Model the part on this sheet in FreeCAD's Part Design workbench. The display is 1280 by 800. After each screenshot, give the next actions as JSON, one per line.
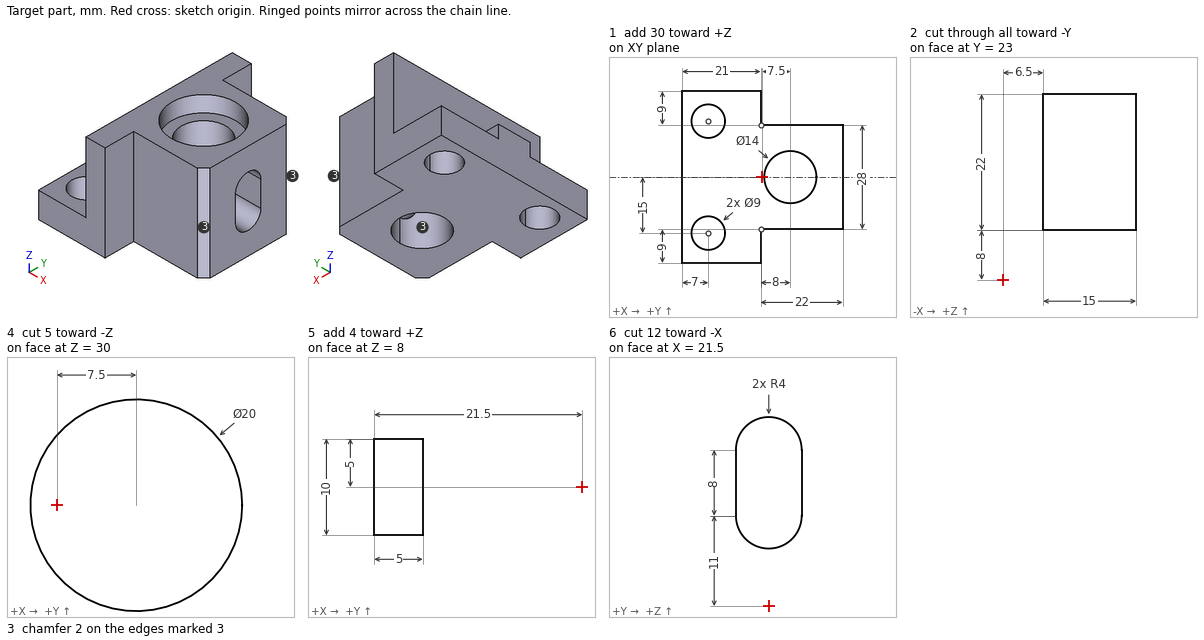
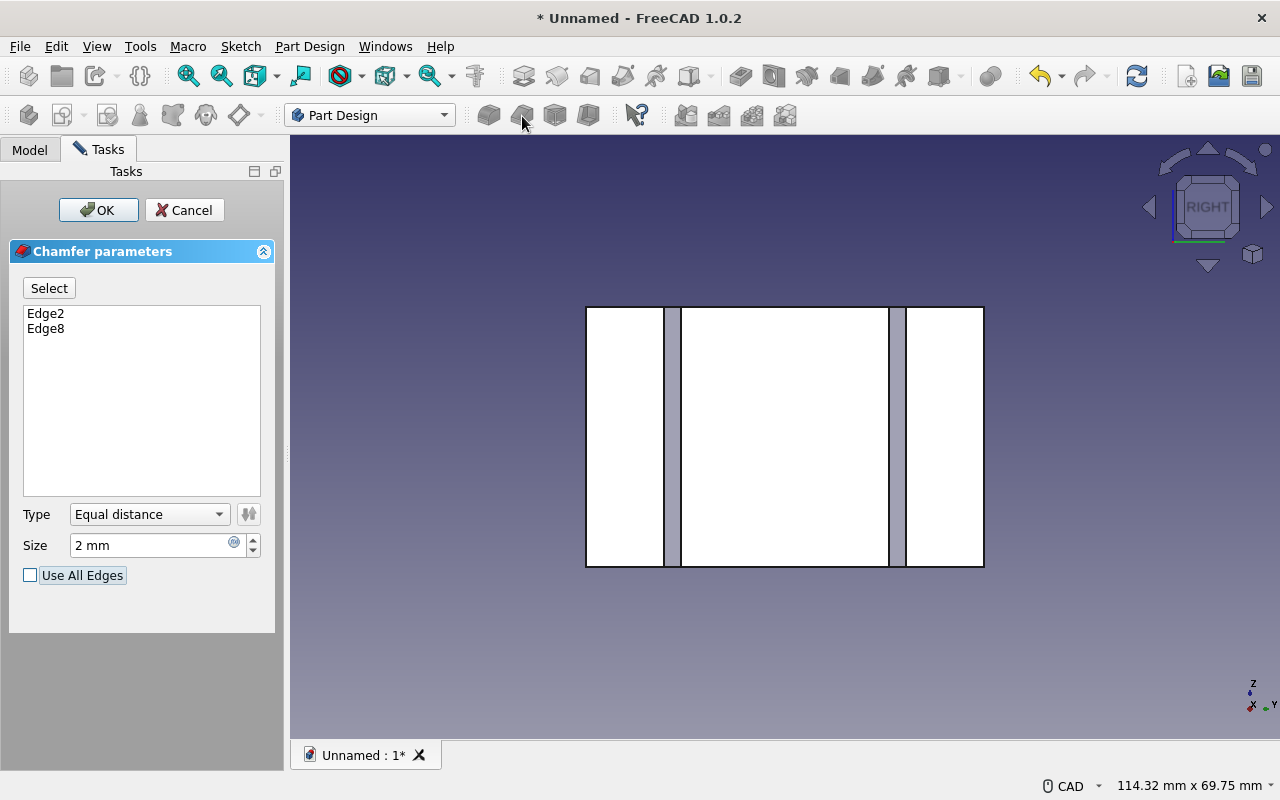
{"action": "left_click", "coordinate": [99, 210]}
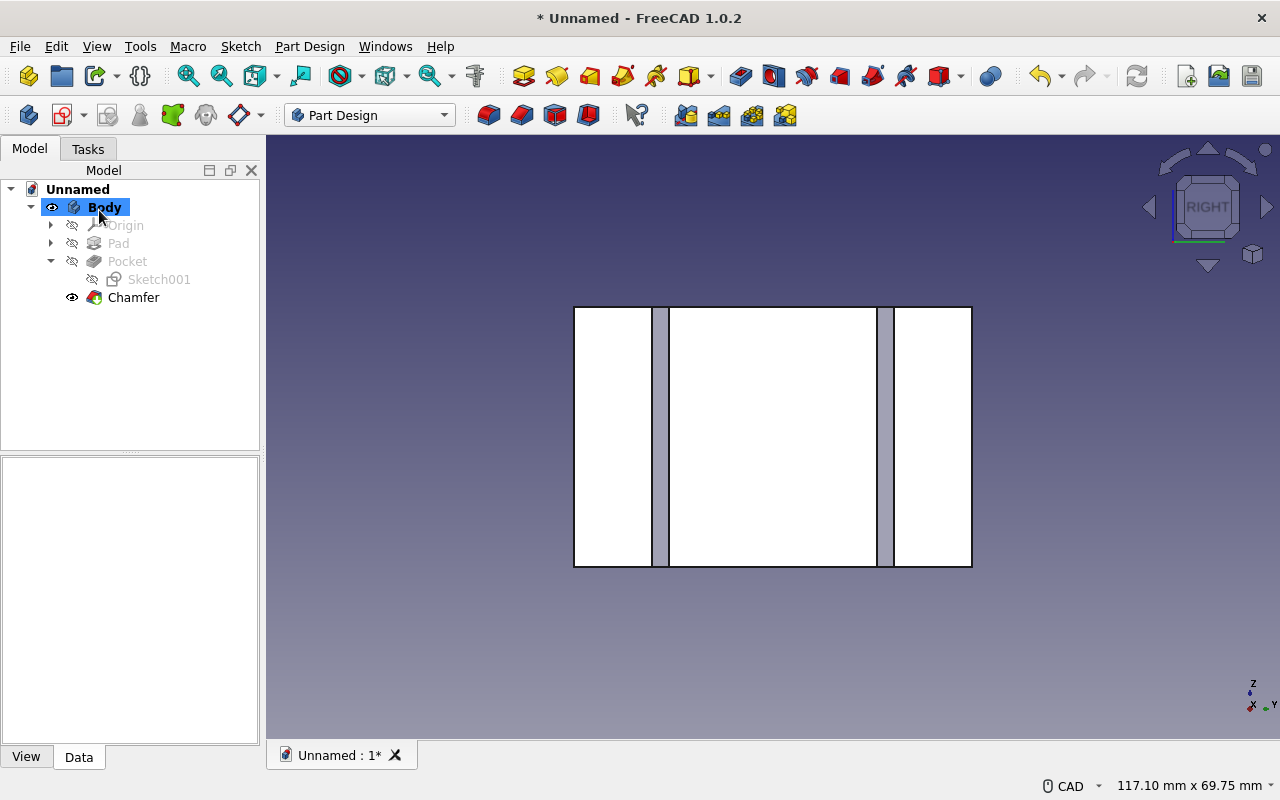
{"action": "key", "text": "v f"}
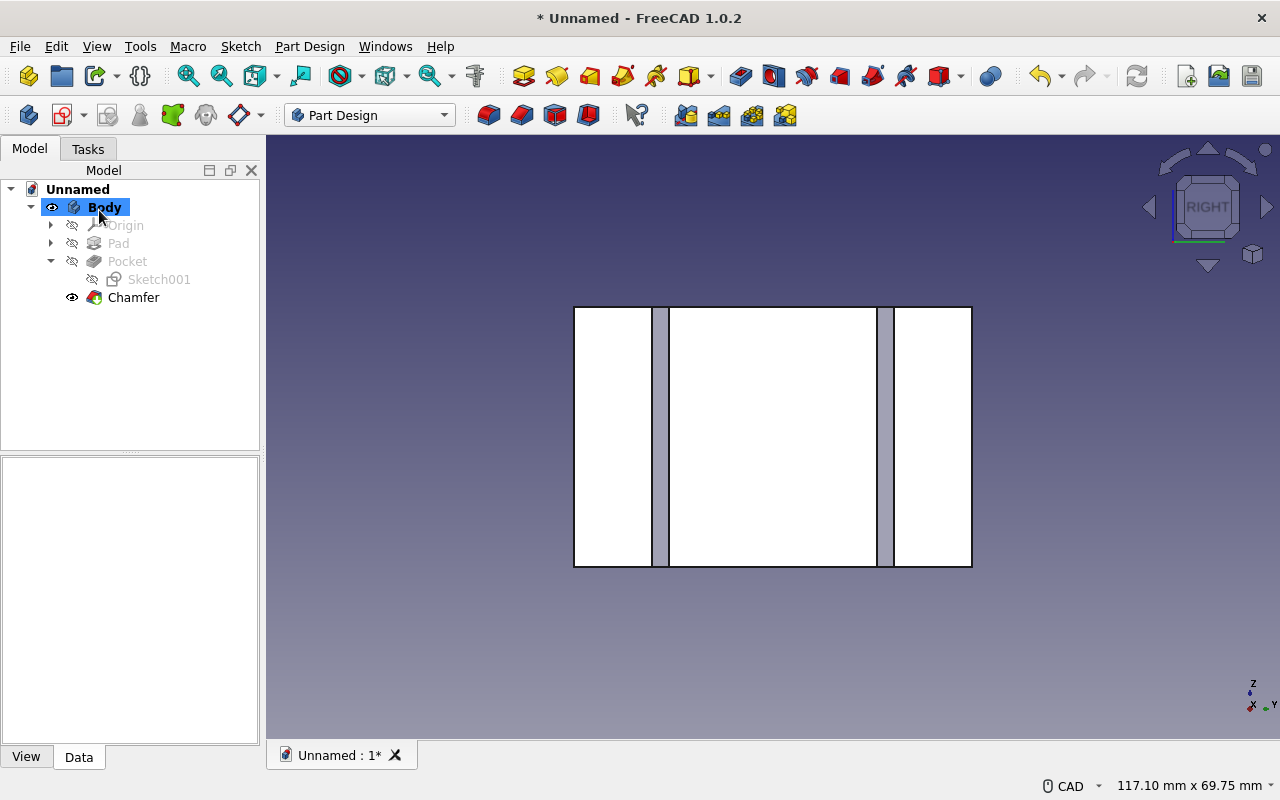
{"action": "key", "text": "0"}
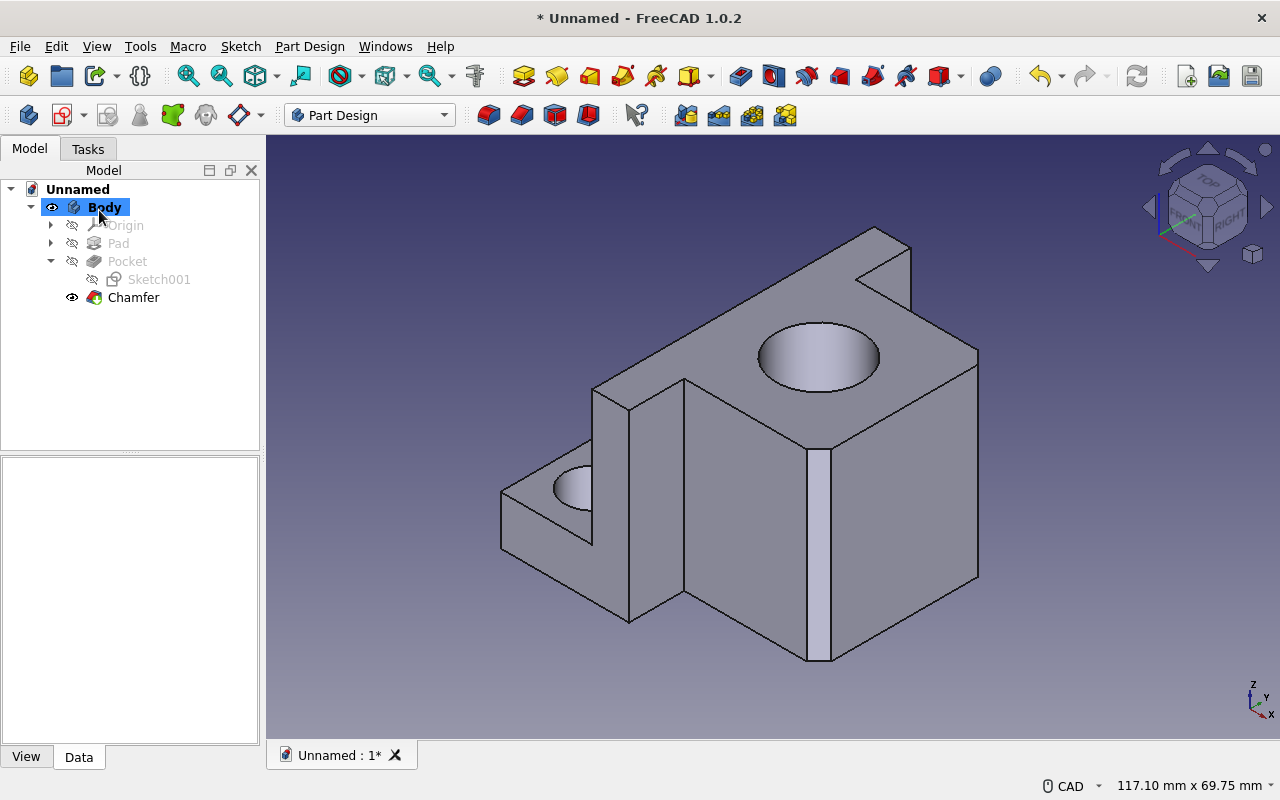
{"action": "left_click", "coordinate": [908, 362]}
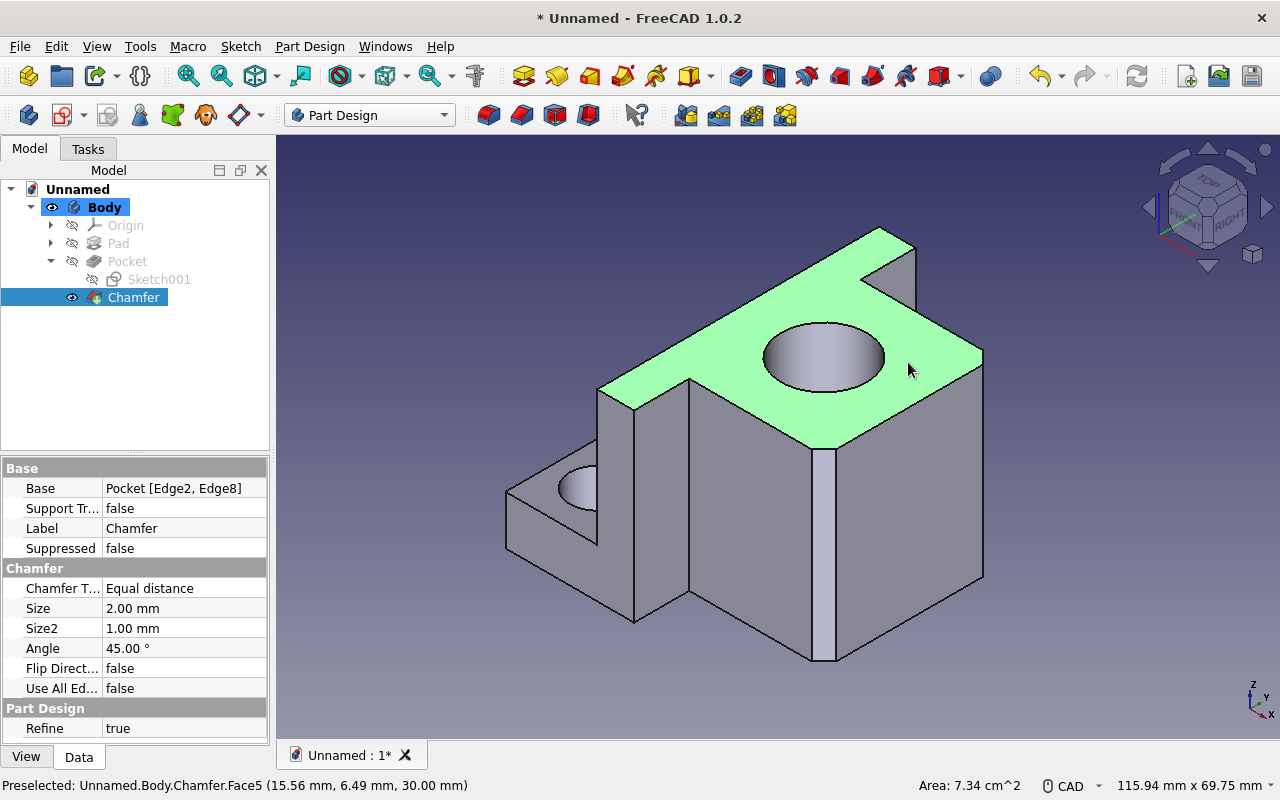
{"action": "left_click", "coordinate": [62, 116]}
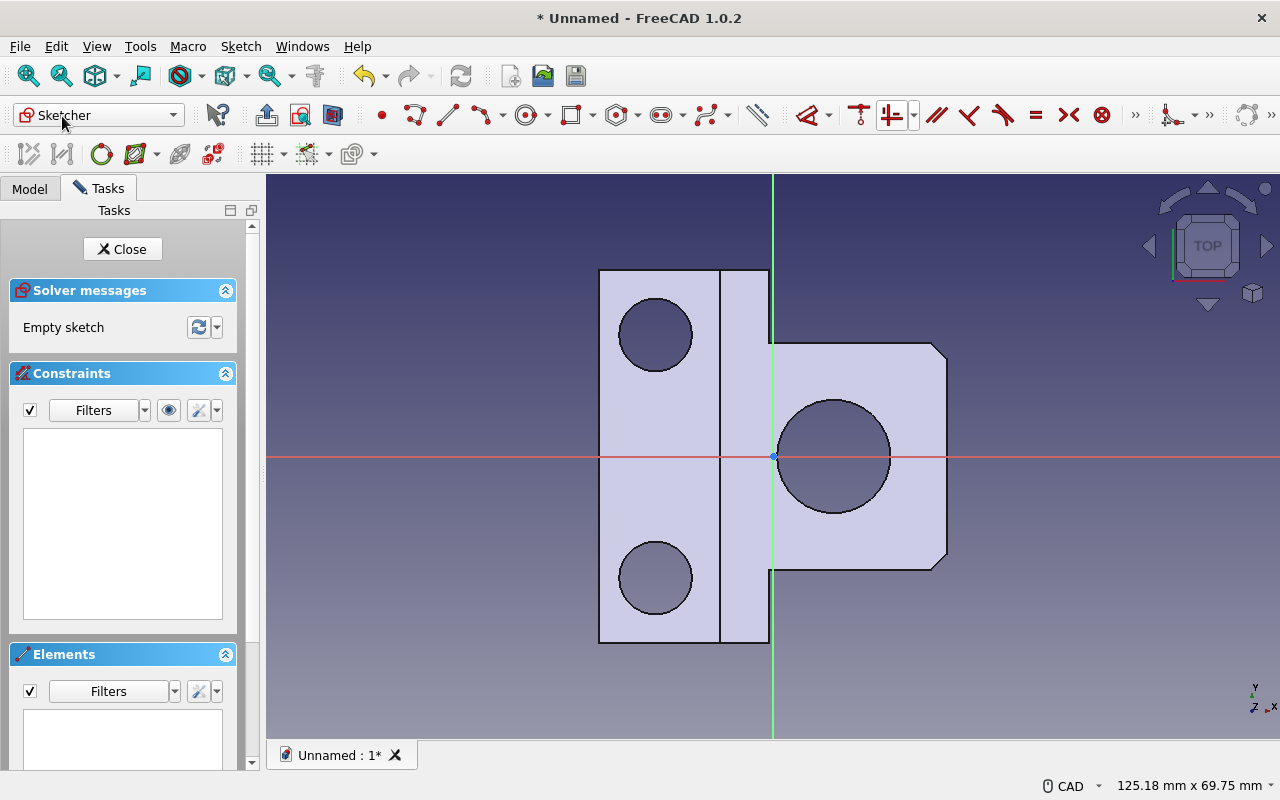
{"action": "scroll", "coordinate": [939, 456], "scroll_direction": "up", "scroll_amount": 4}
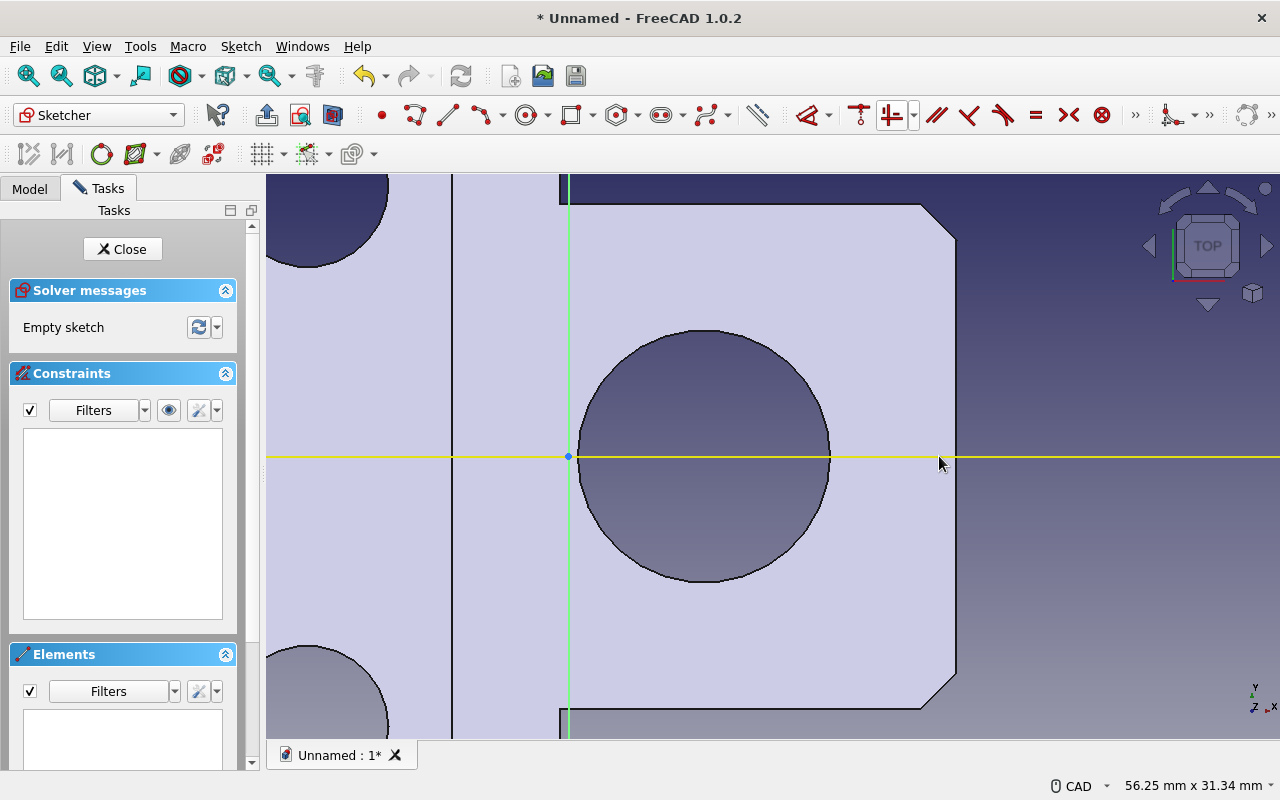
{"action": "key", "text": "g c"}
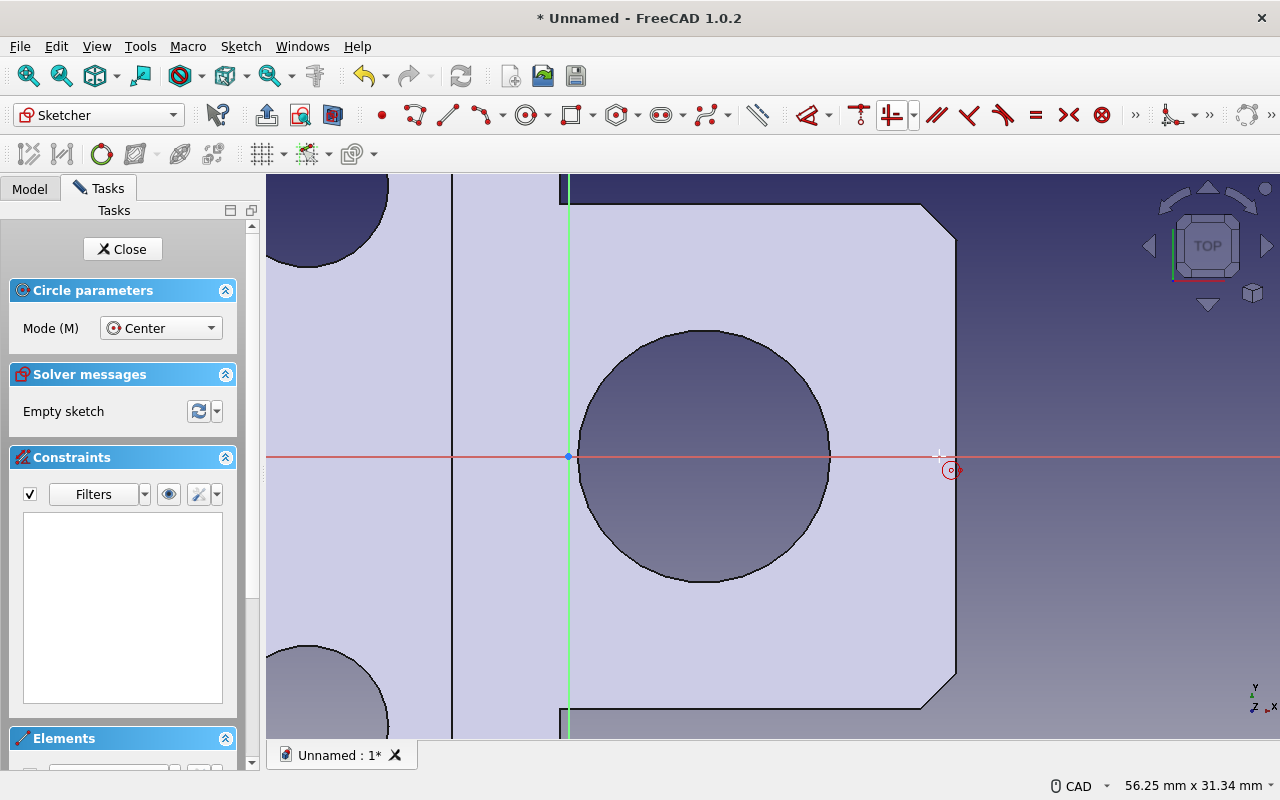
{"action": "left_click", "coordinate": [704, 456]}
{"action": "left_click", "coordinate": [831, 329]}
{"action": "key", "text": "Escape"}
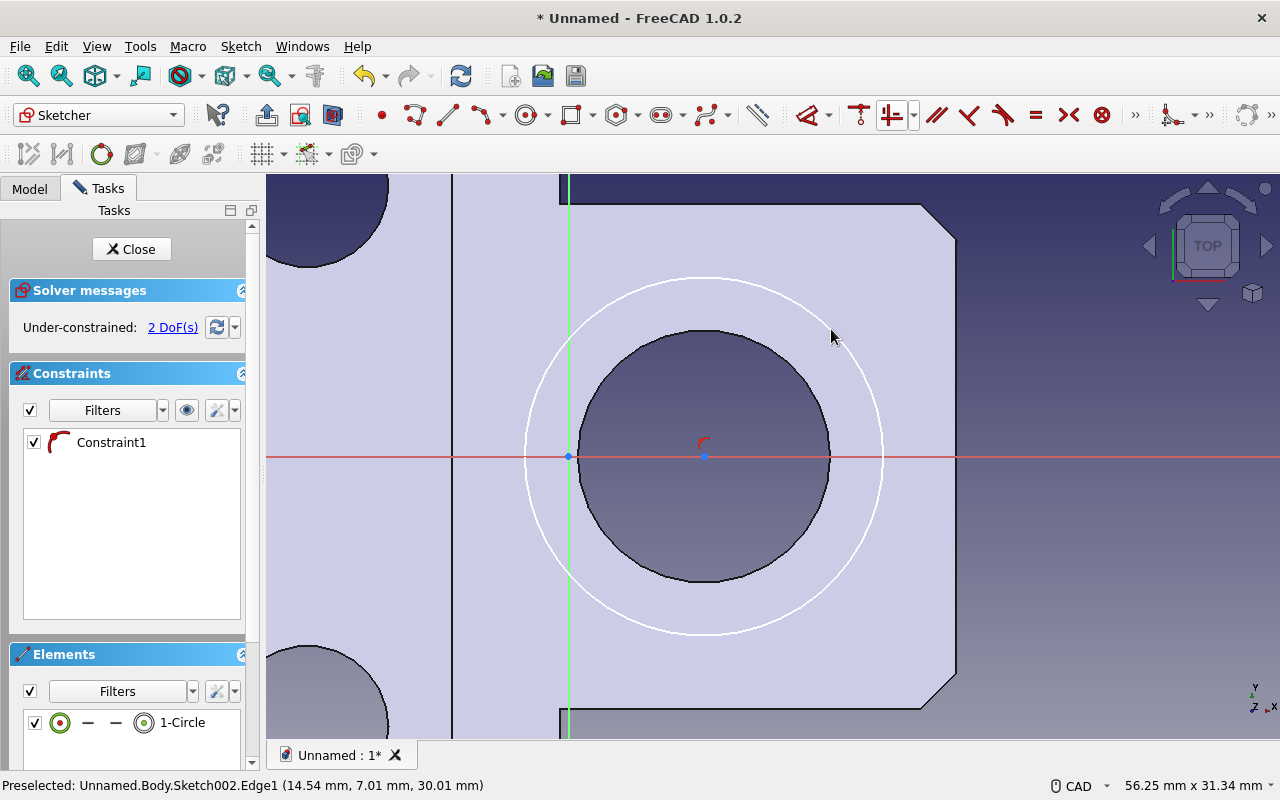
{"action": "key", "text": "d"}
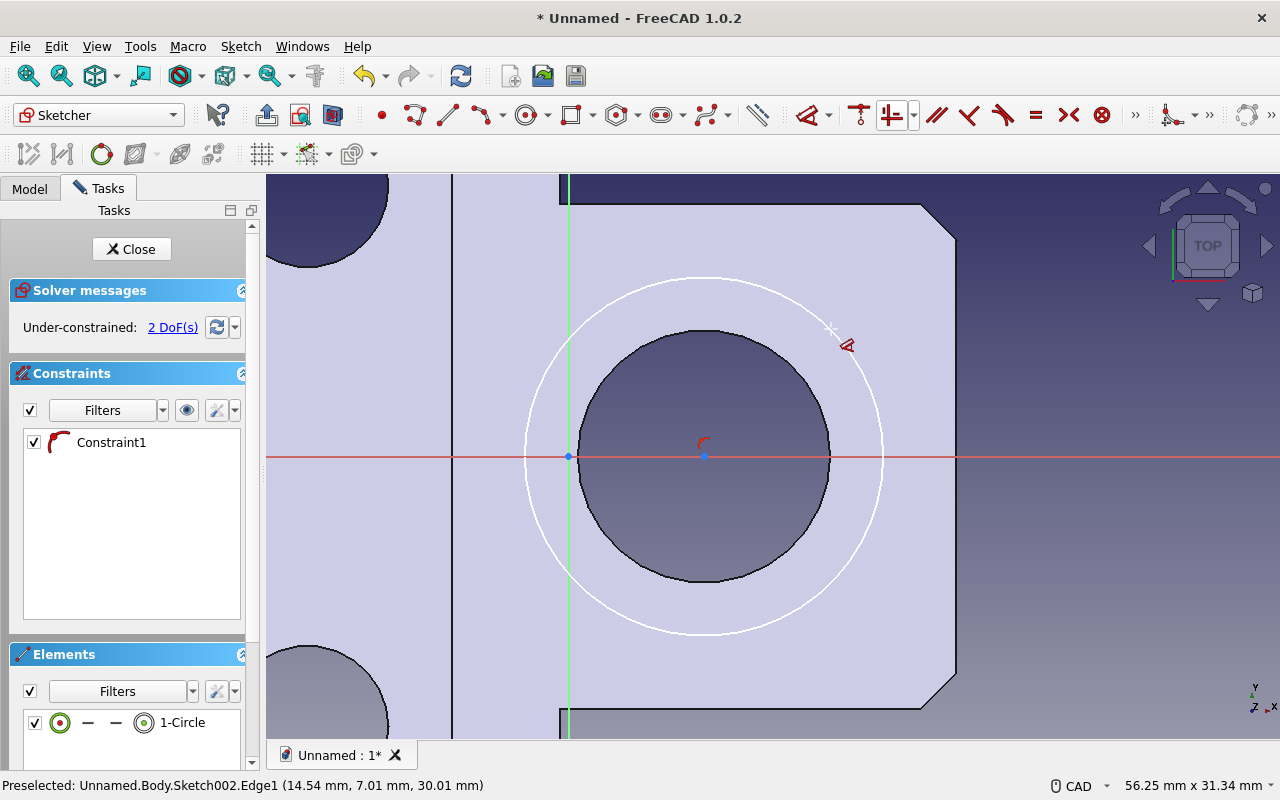
{"action": "left_click", "coordinate": [830, 329]}
{"action": "left_click", "coordinate": [852, 306]}